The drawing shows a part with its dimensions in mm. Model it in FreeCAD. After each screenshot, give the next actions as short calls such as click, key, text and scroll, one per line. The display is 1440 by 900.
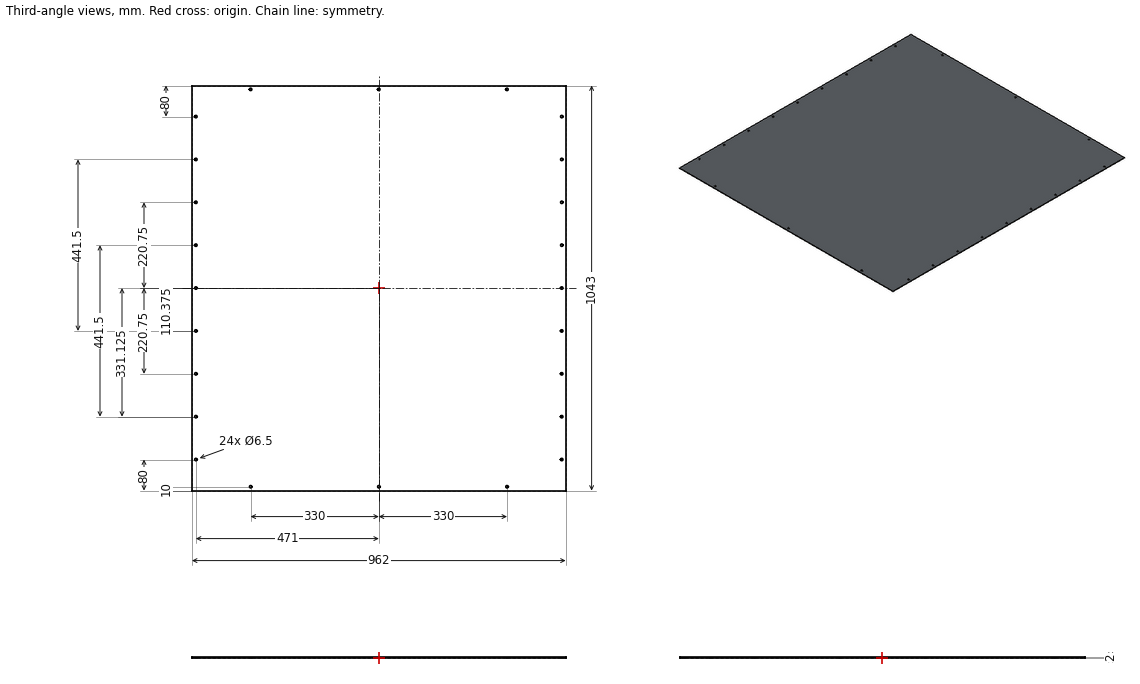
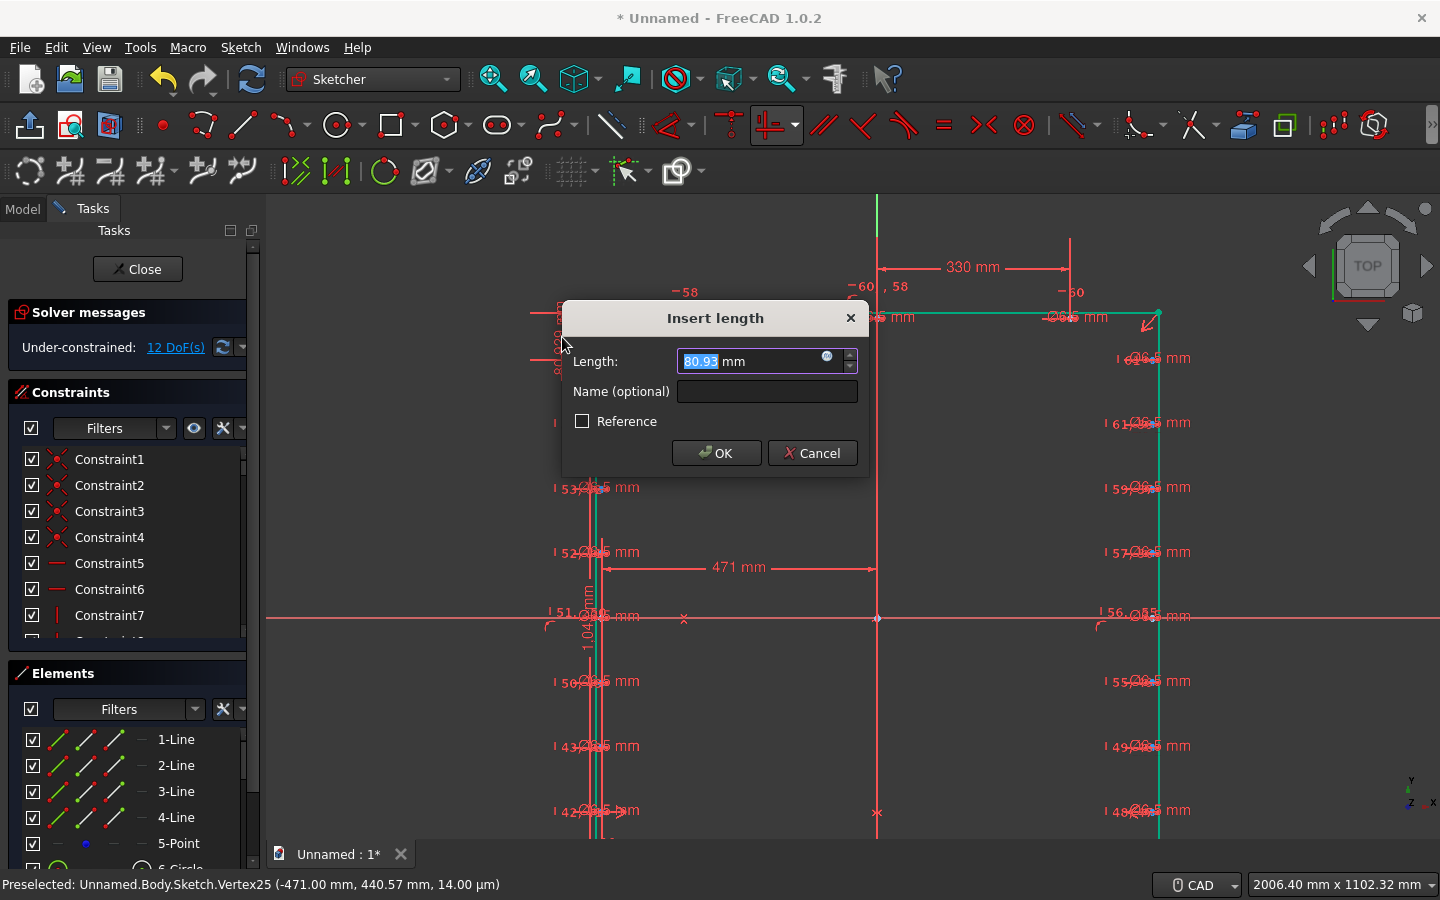
text(80)
key(Return)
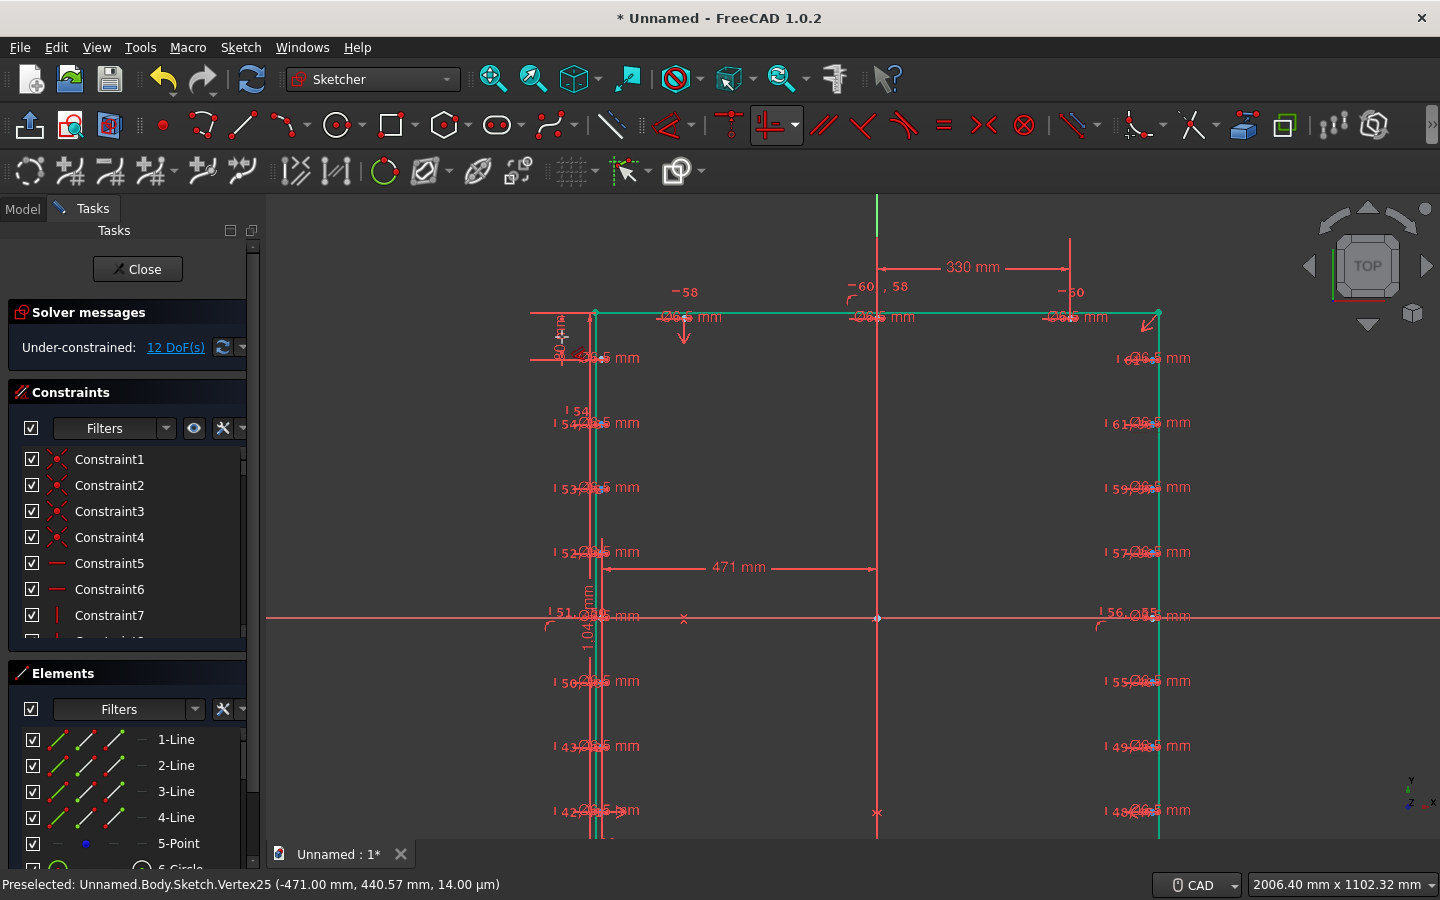
click(1159, 313)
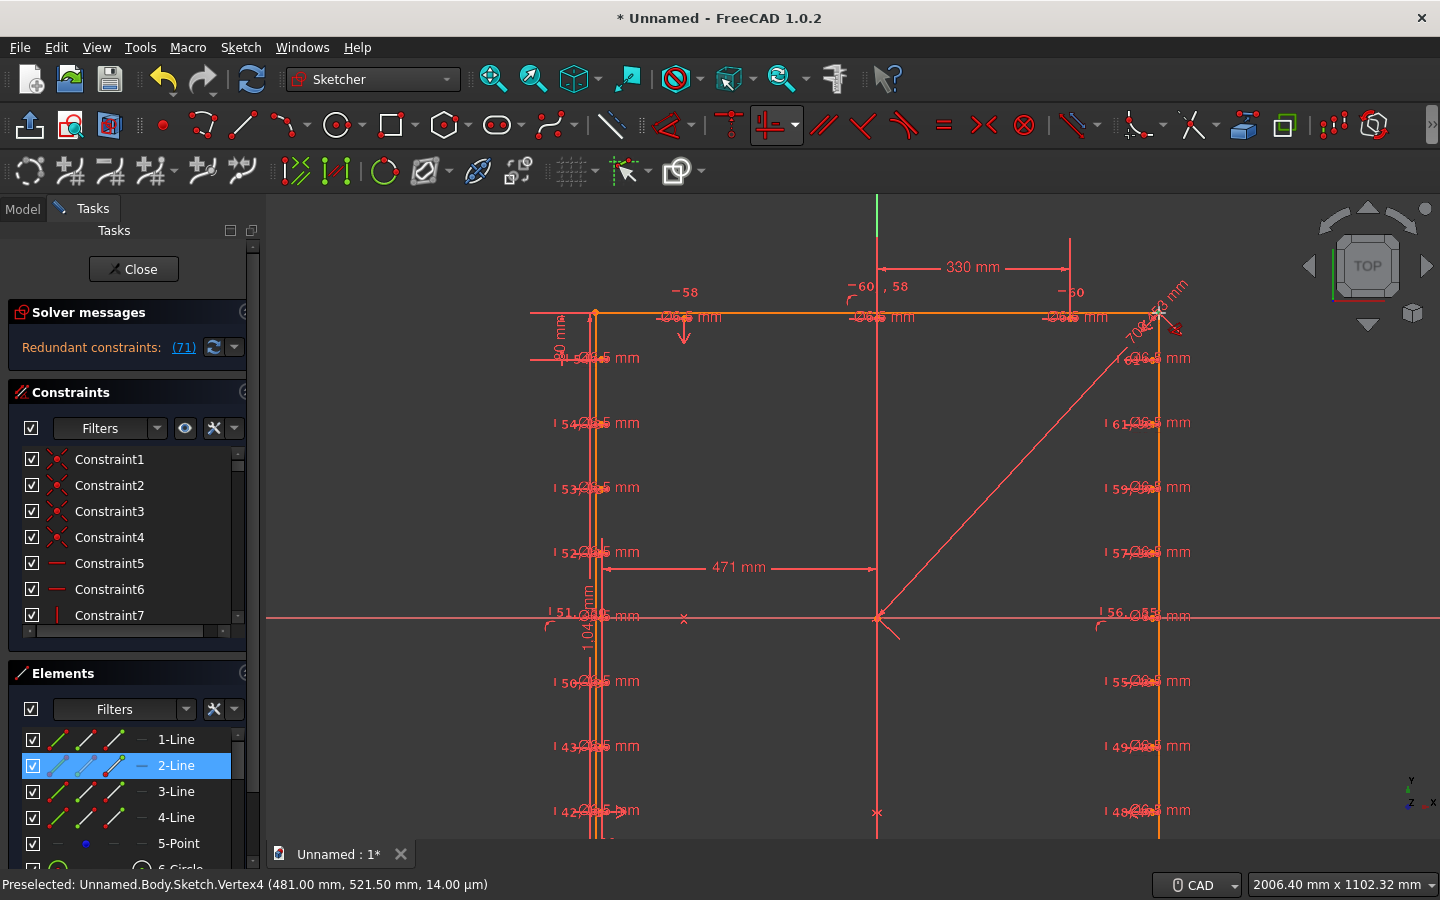
click(1153, 360)
click(1193, 336)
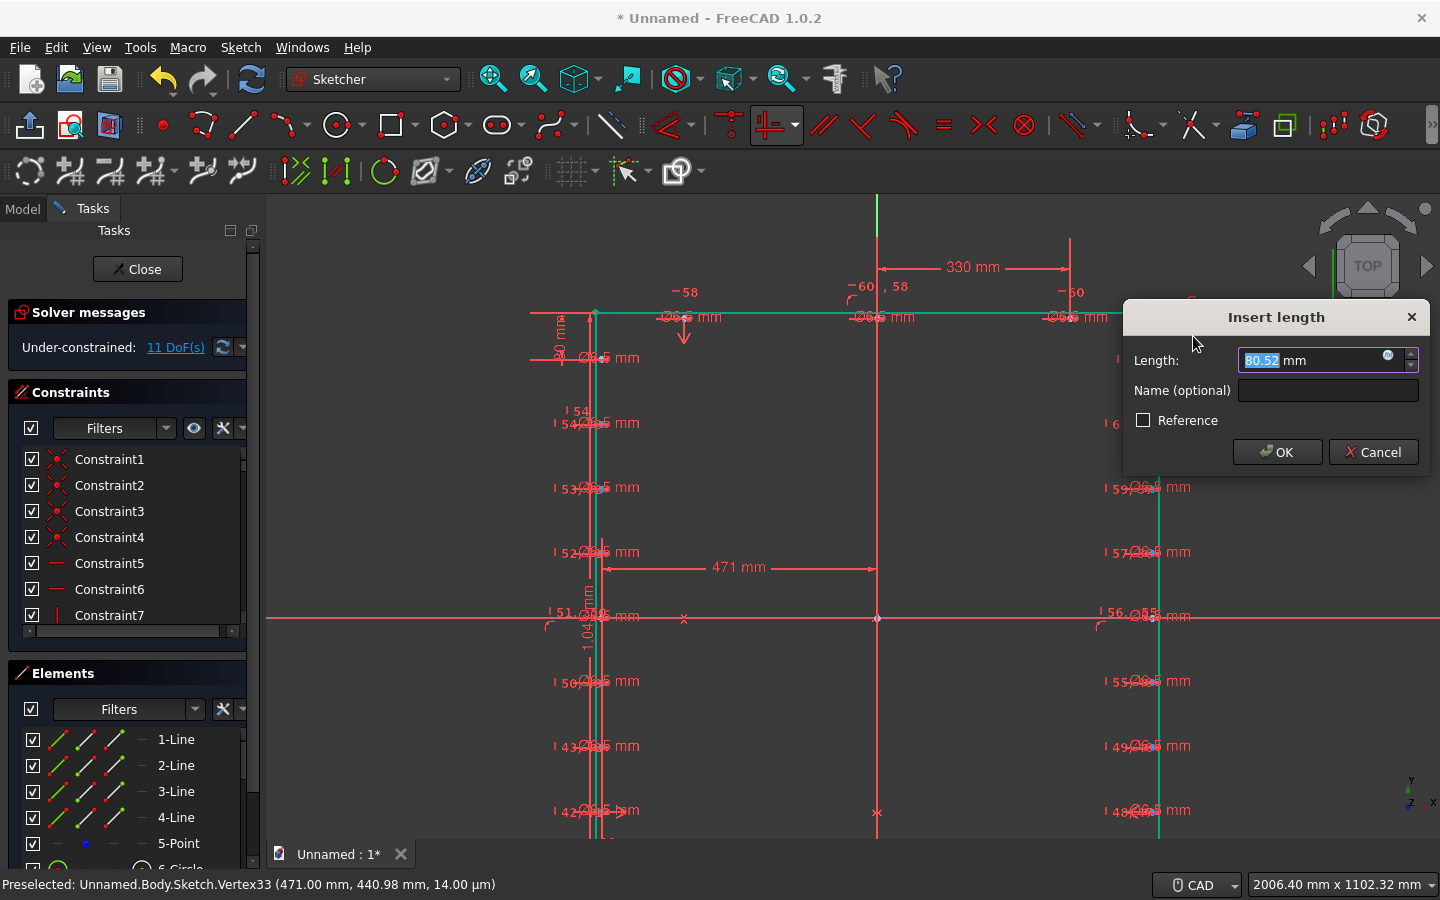
text(80)
key(Return)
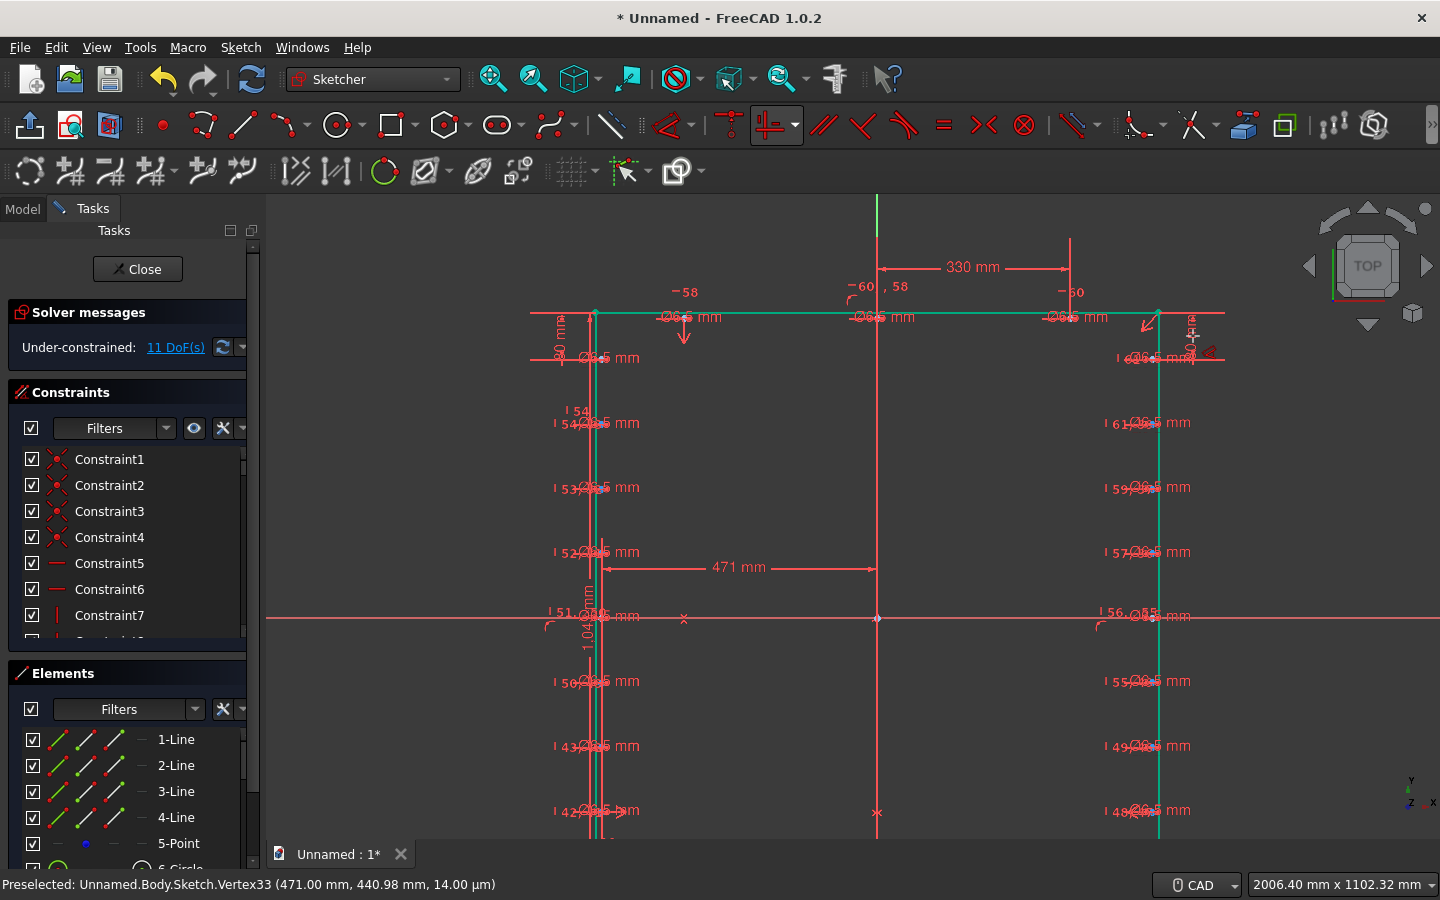
click(602, 748)
click(568, 683)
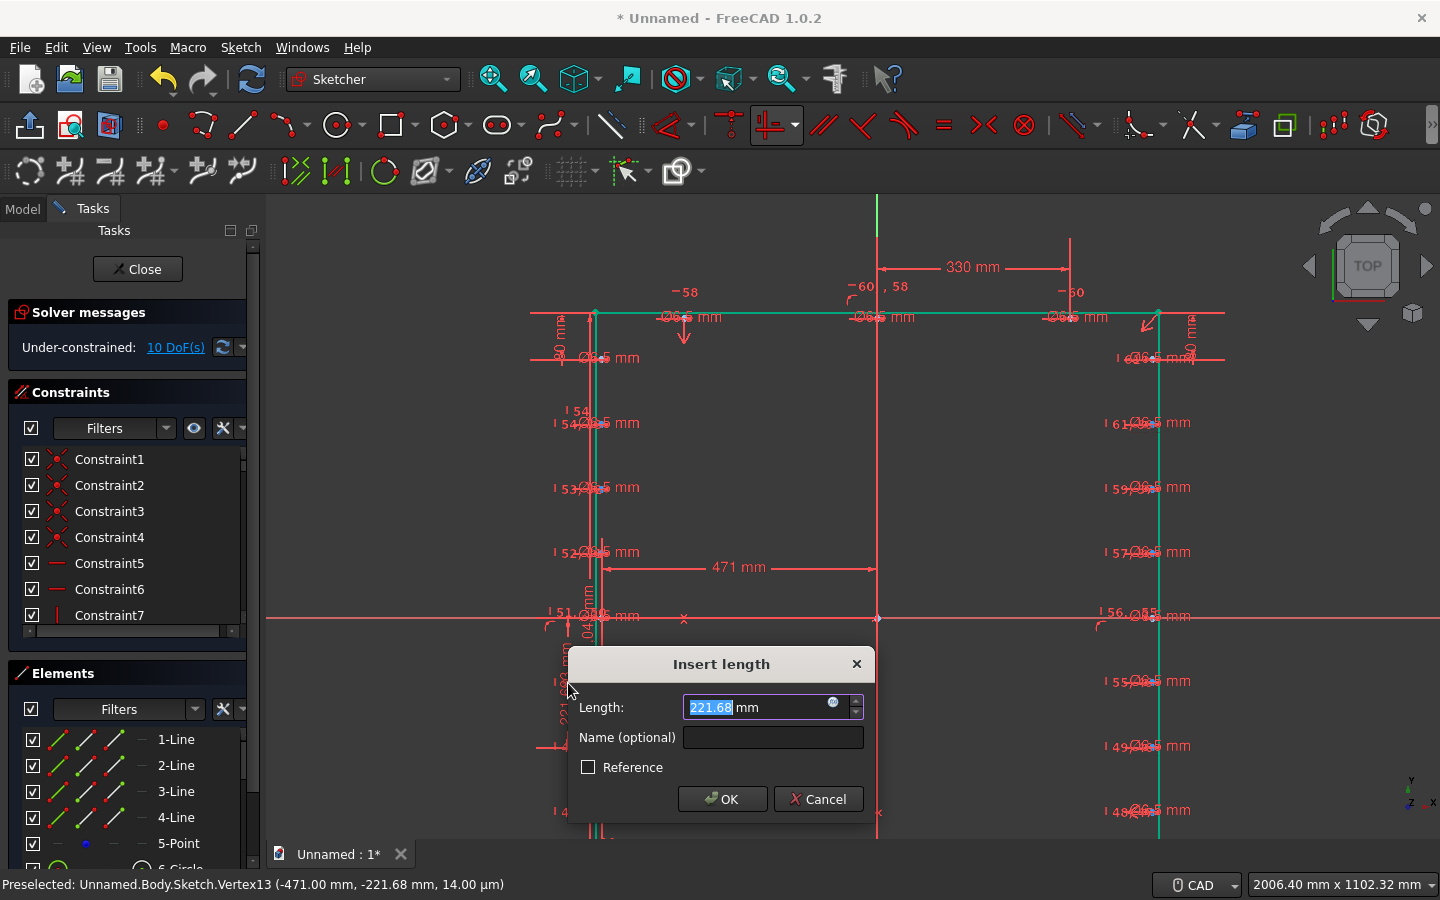
text(220.75)
key(Return)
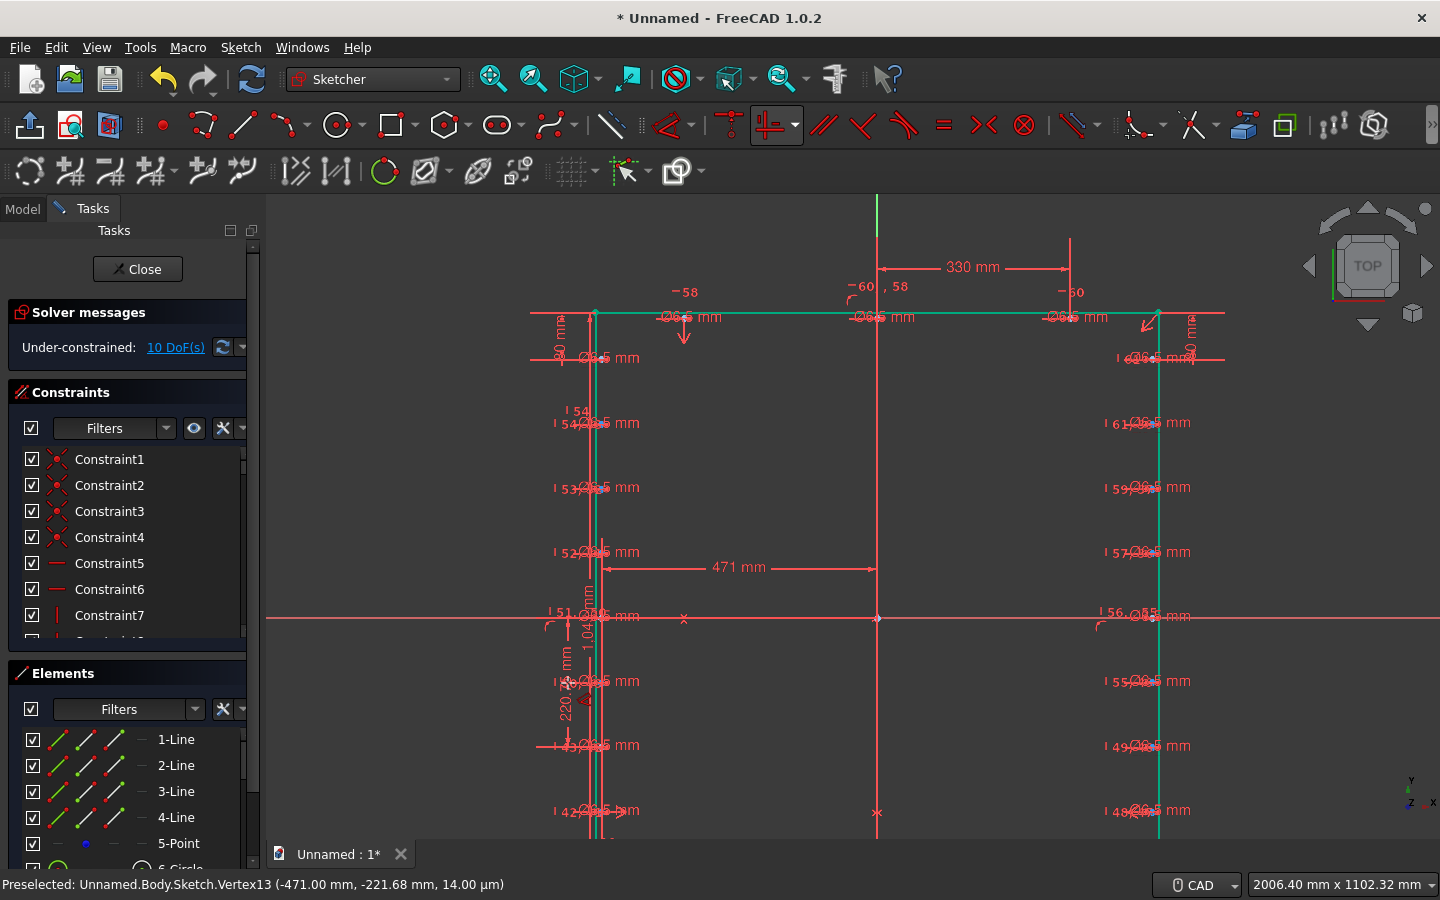
click(1153, 748)
click(1187, 683)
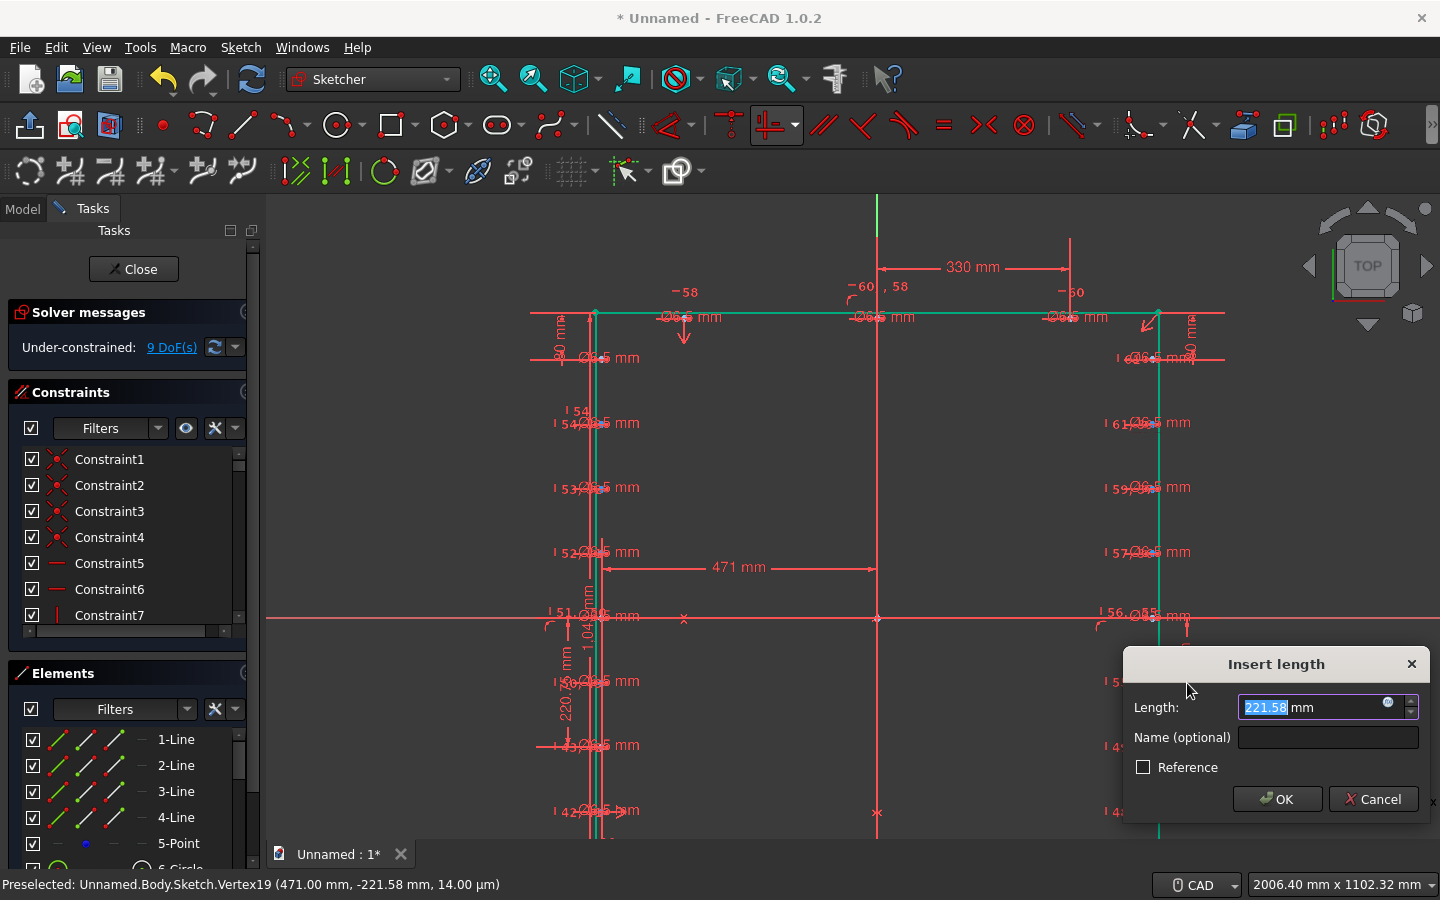
text(220.75)
key(Return)